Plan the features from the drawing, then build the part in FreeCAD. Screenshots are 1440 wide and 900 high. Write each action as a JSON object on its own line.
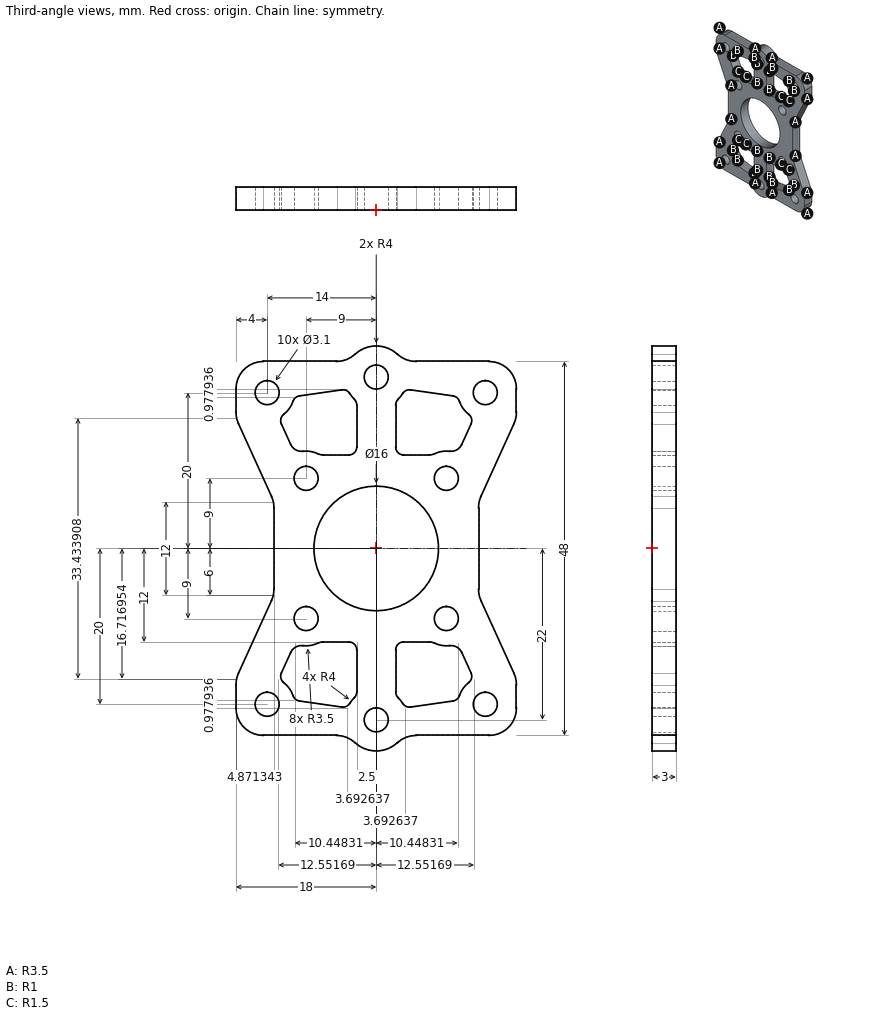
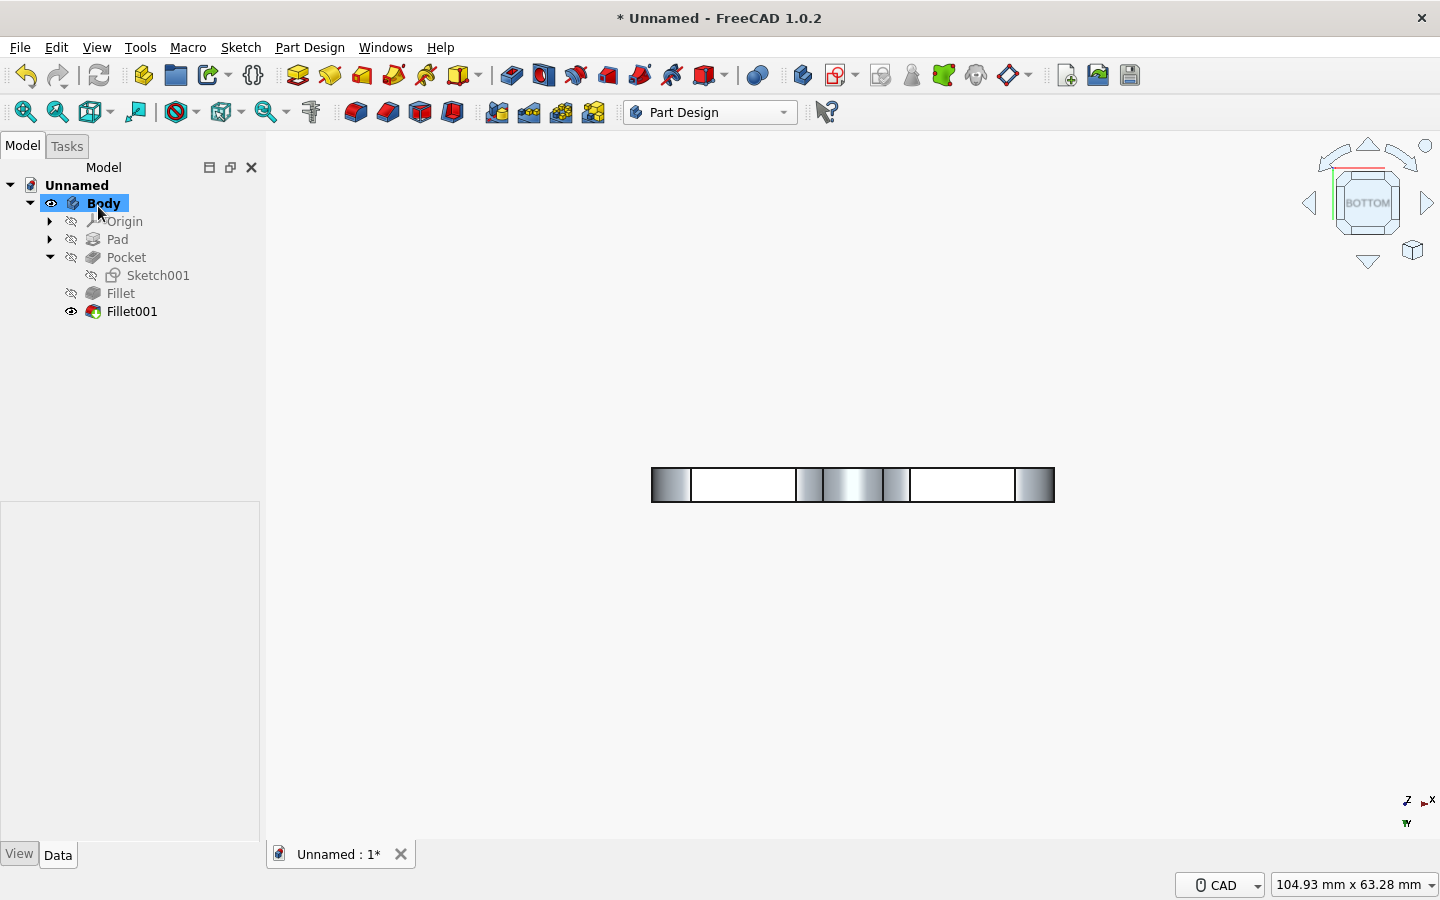
{"action": "key", "text": "v f"}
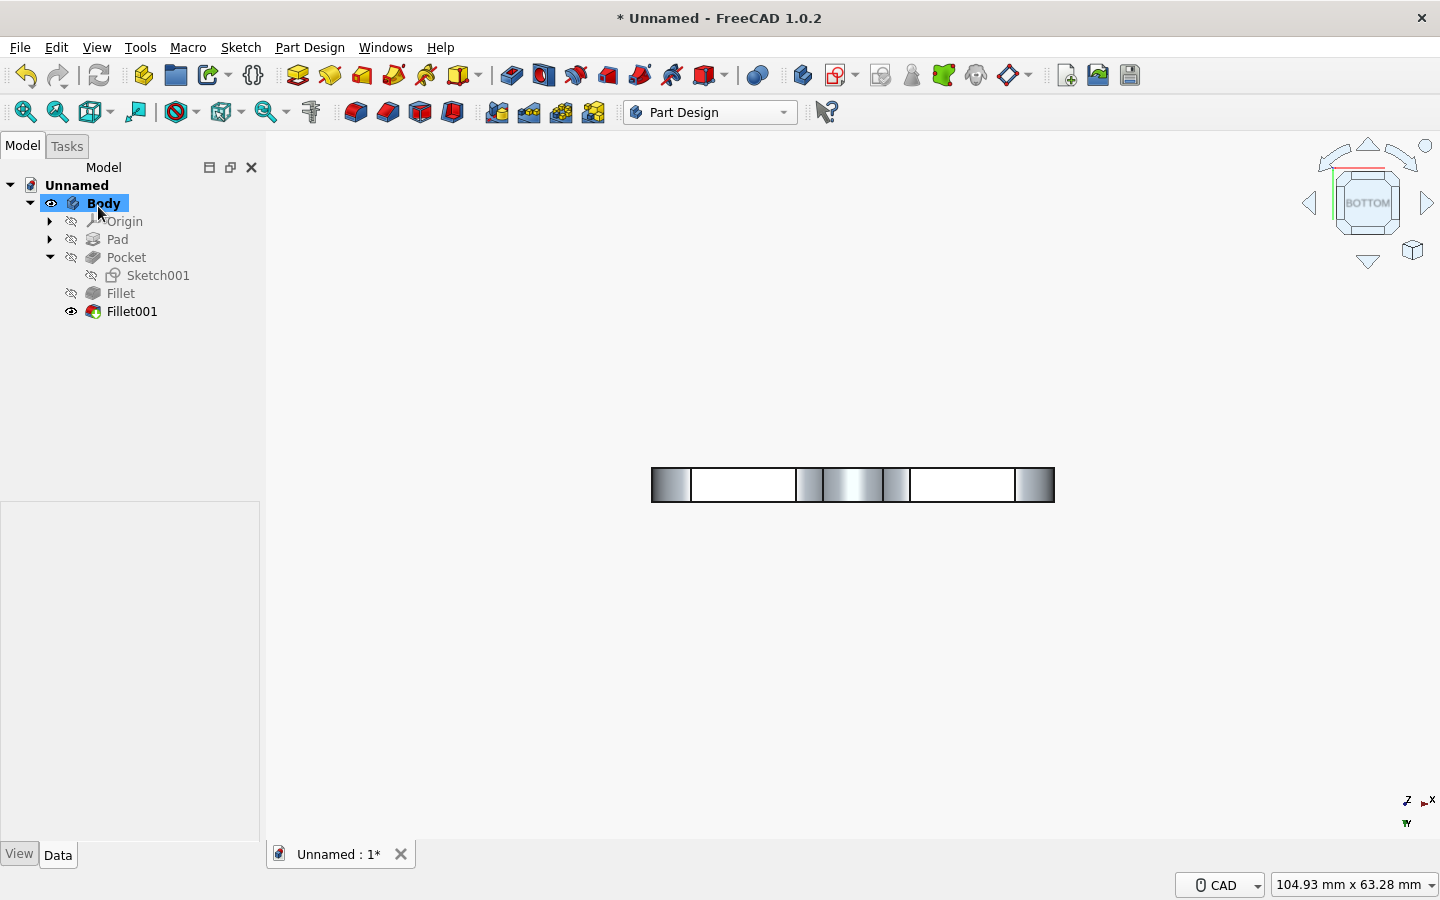
{"action": "key", "text": "4"}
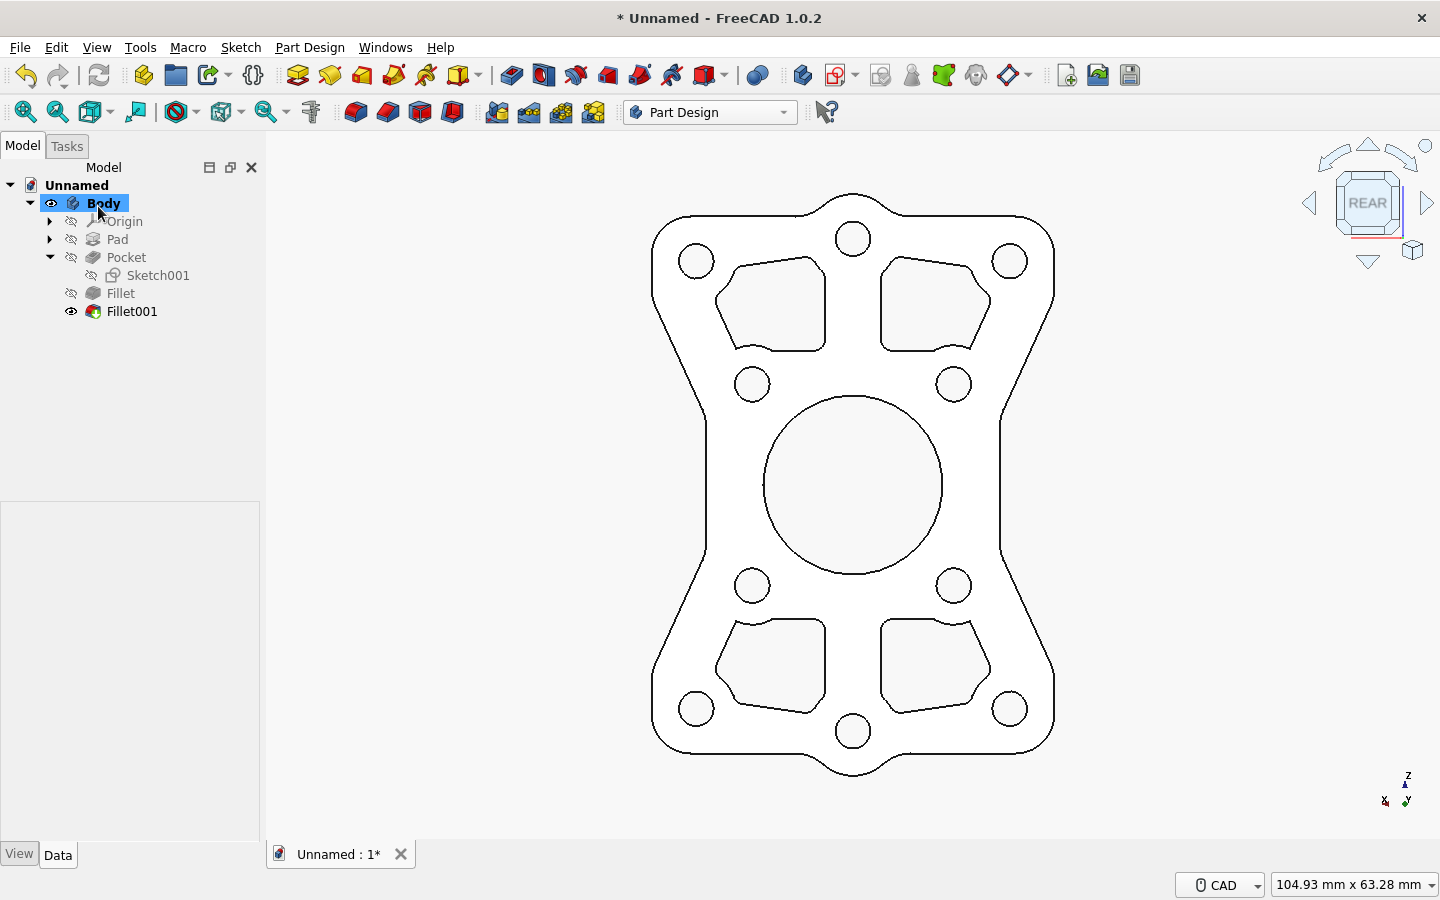
{"action": "key", "text": "6"}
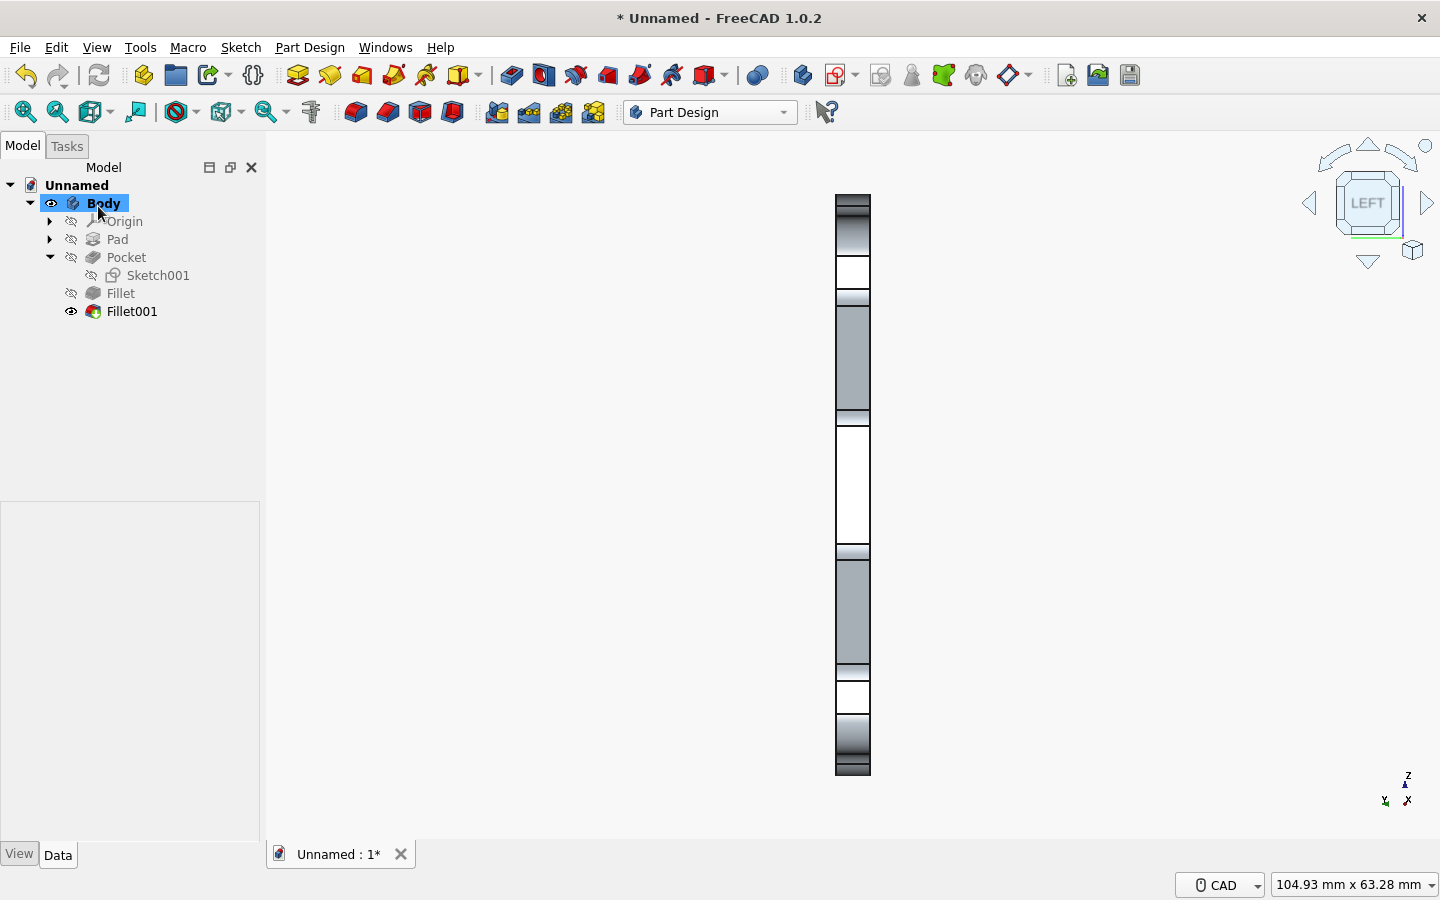
{"action": "key", "text": "v 3"}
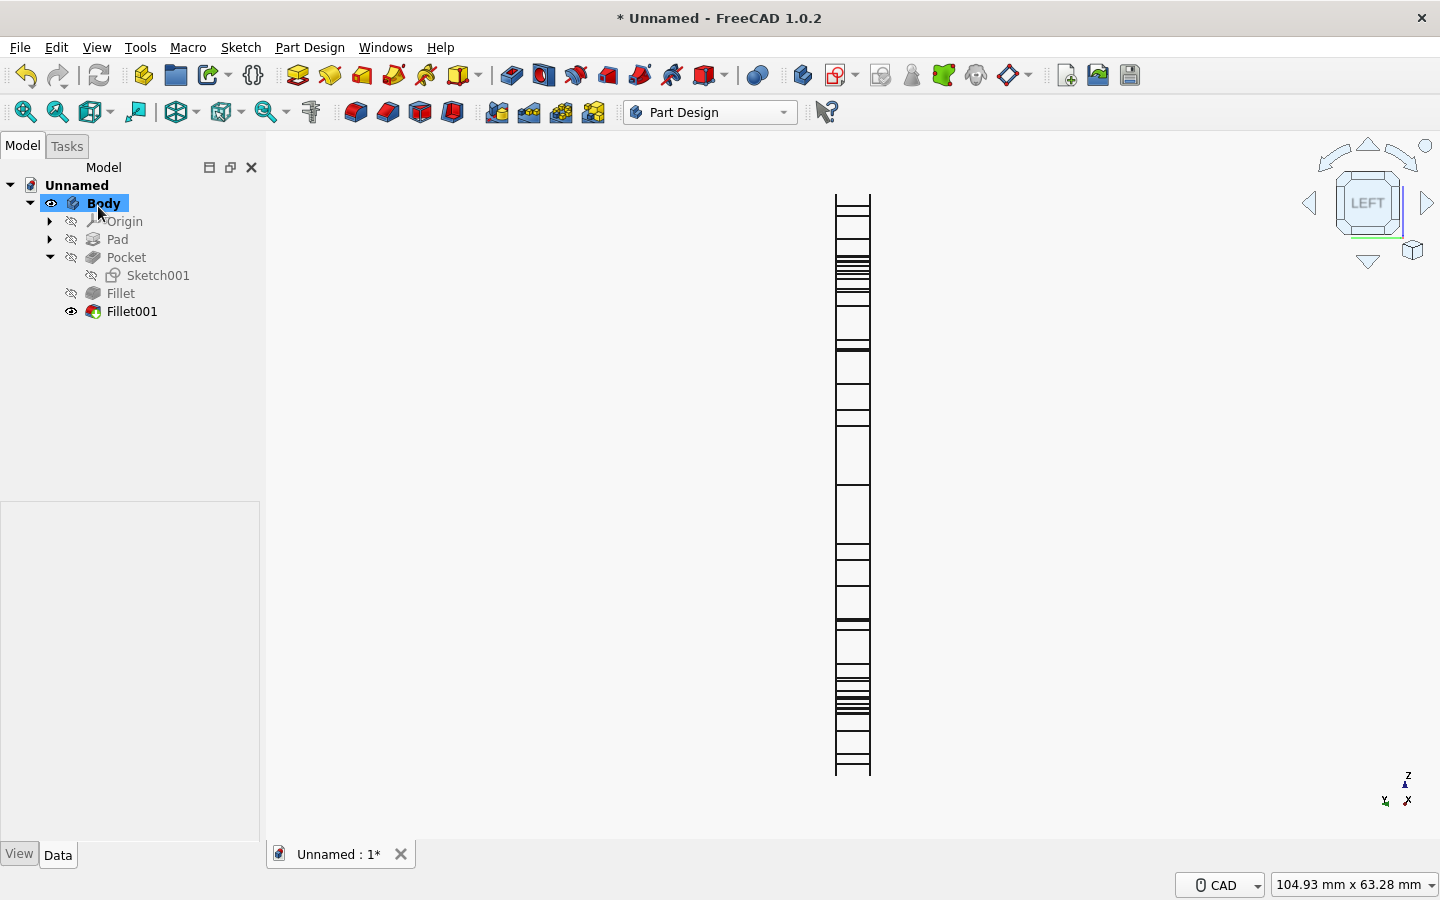
{"action": "key", "text": "0"}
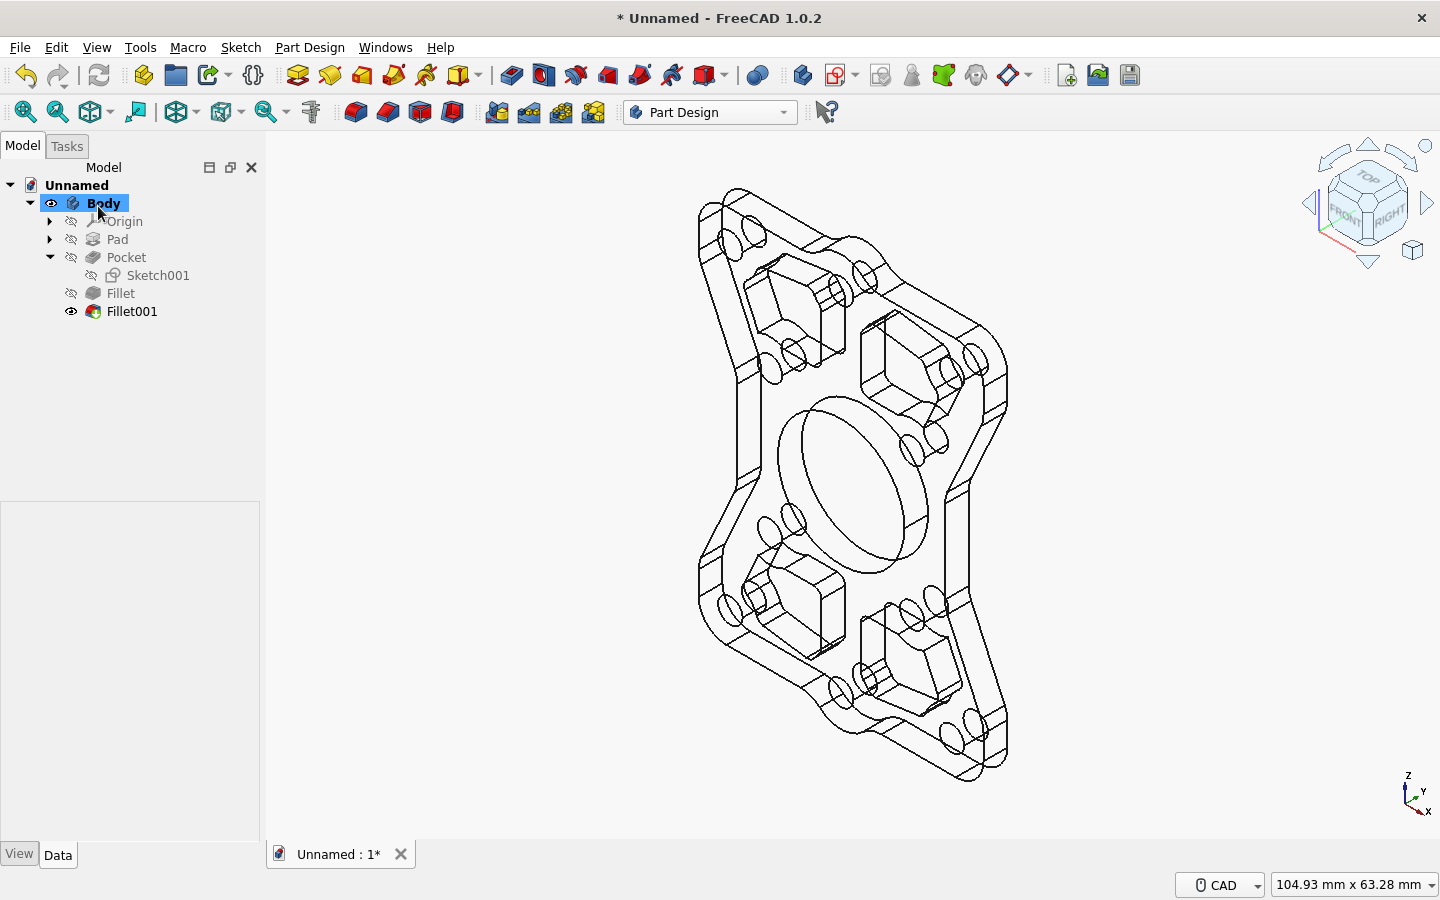
{"action": "left_click", "coordinate": [770, 325]}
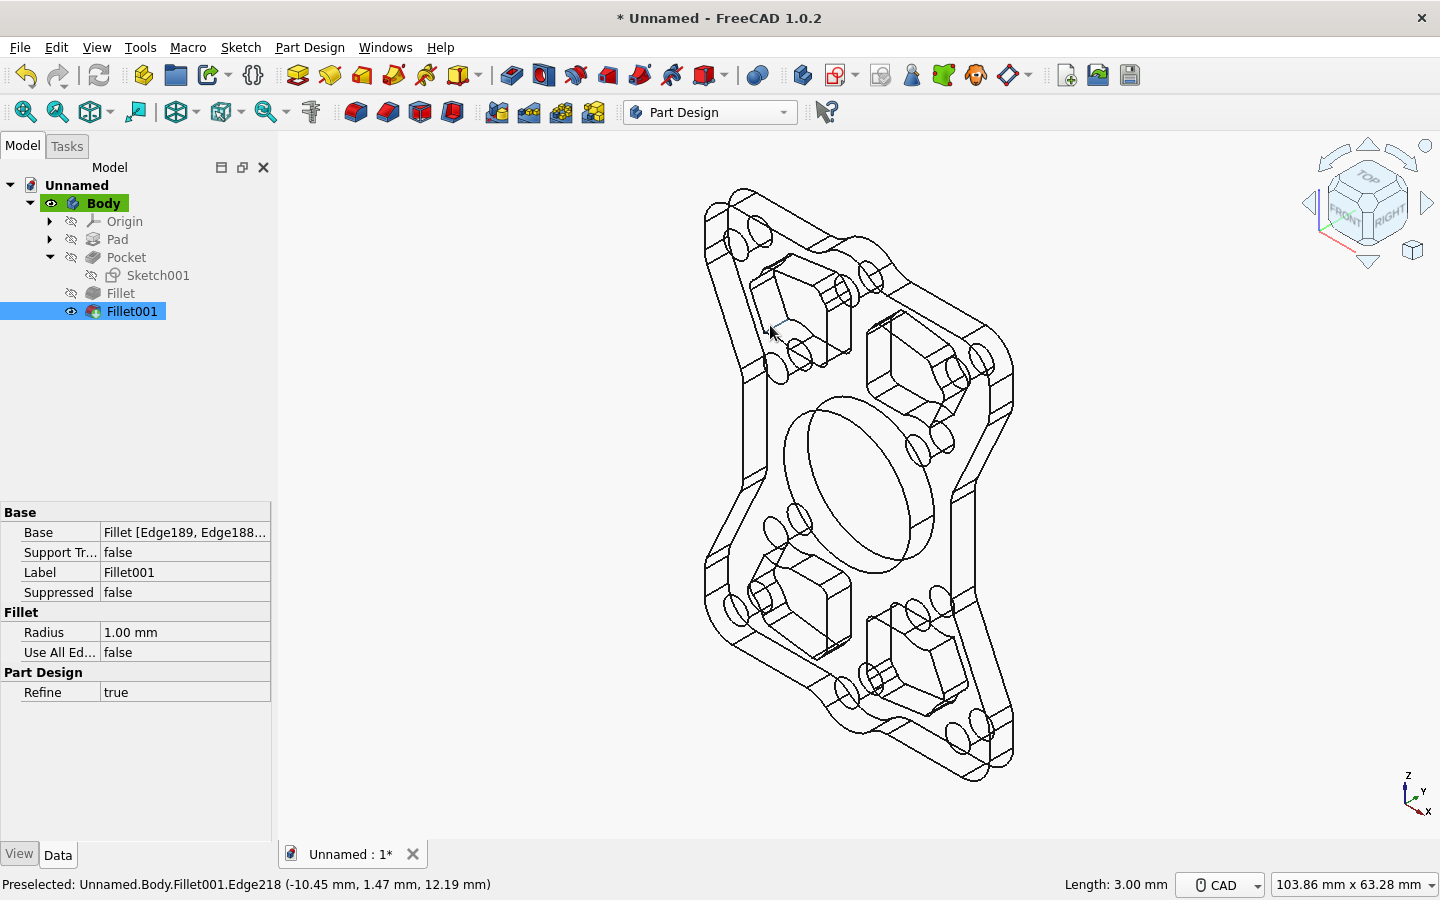
{"action": "left_click", "coordinate": [802, 342], "text": "ctrl"}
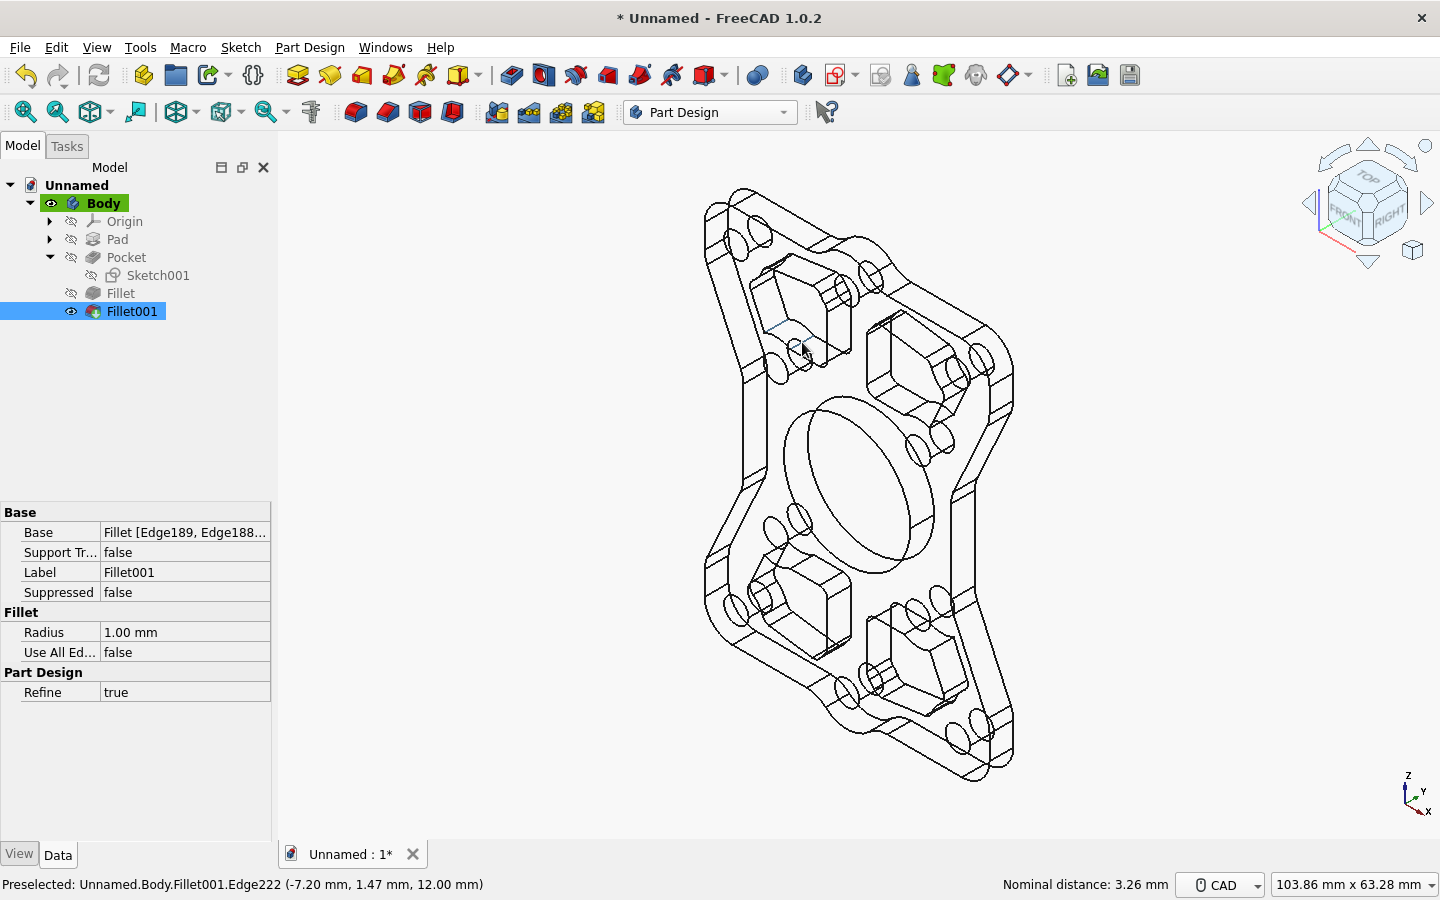
{"action": "left_click", "coordinate": [942, 643], "text": "ctrl"}